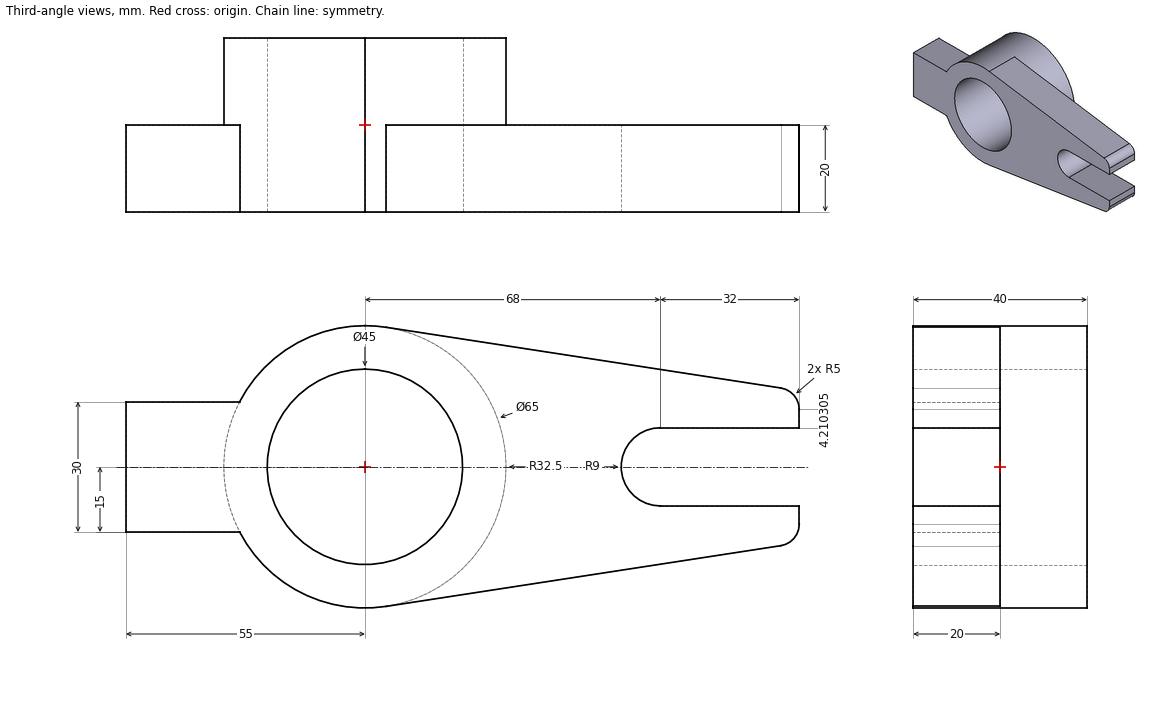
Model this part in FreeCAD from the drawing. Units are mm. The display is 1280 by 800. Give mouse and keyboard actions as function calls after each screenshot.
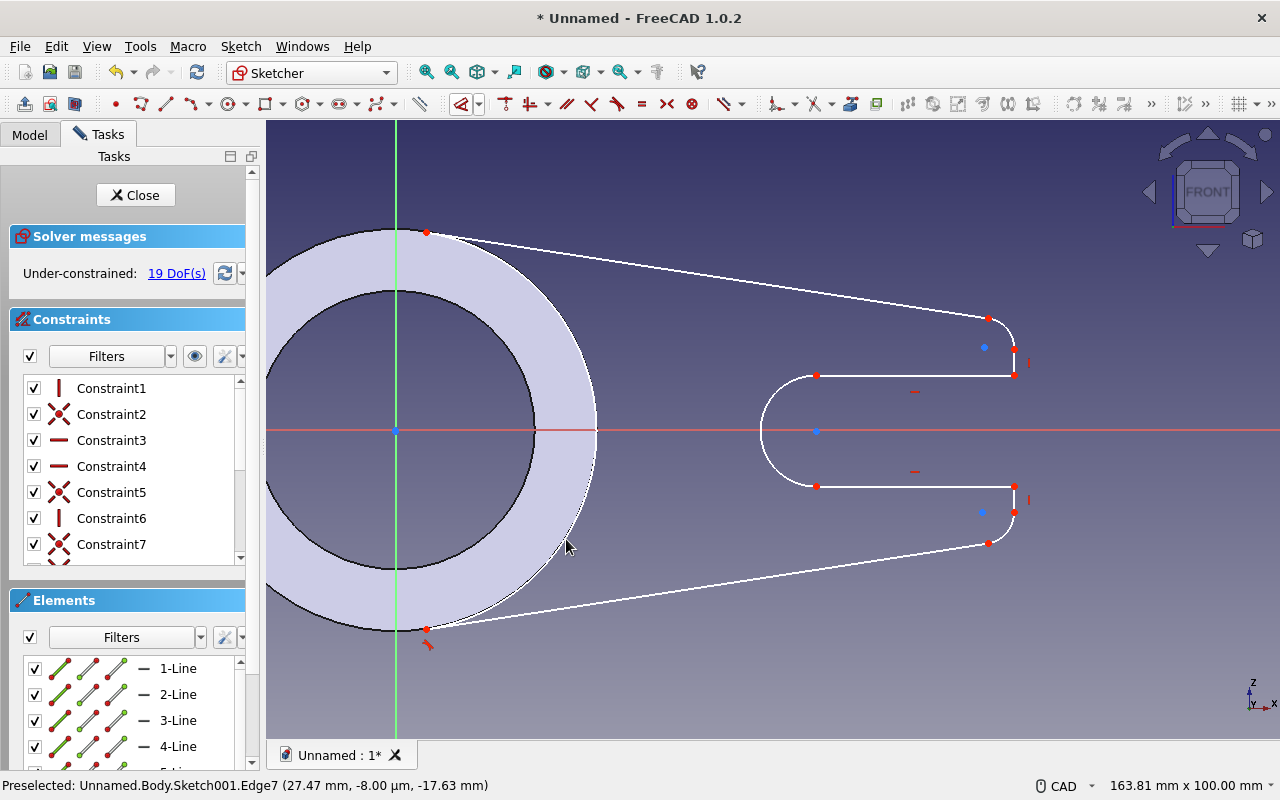
click(820, 569)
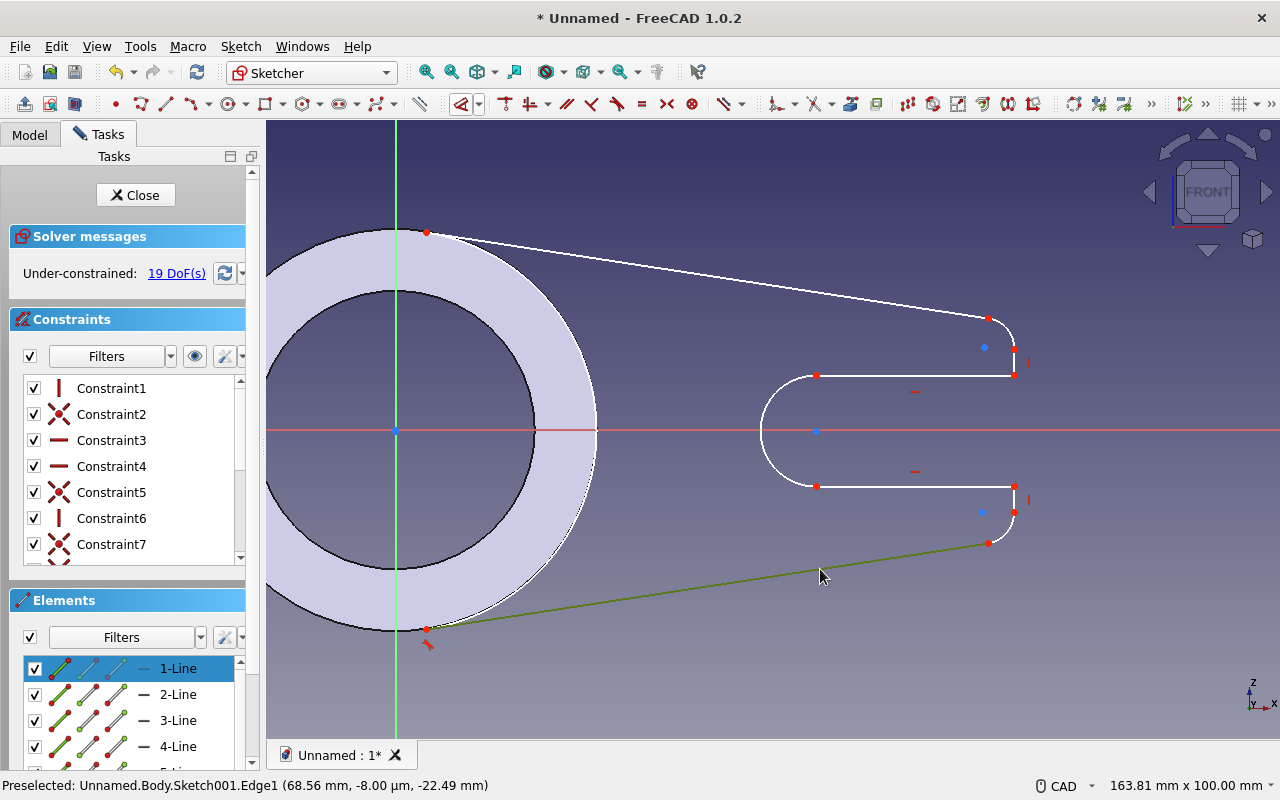
click(1000, 539)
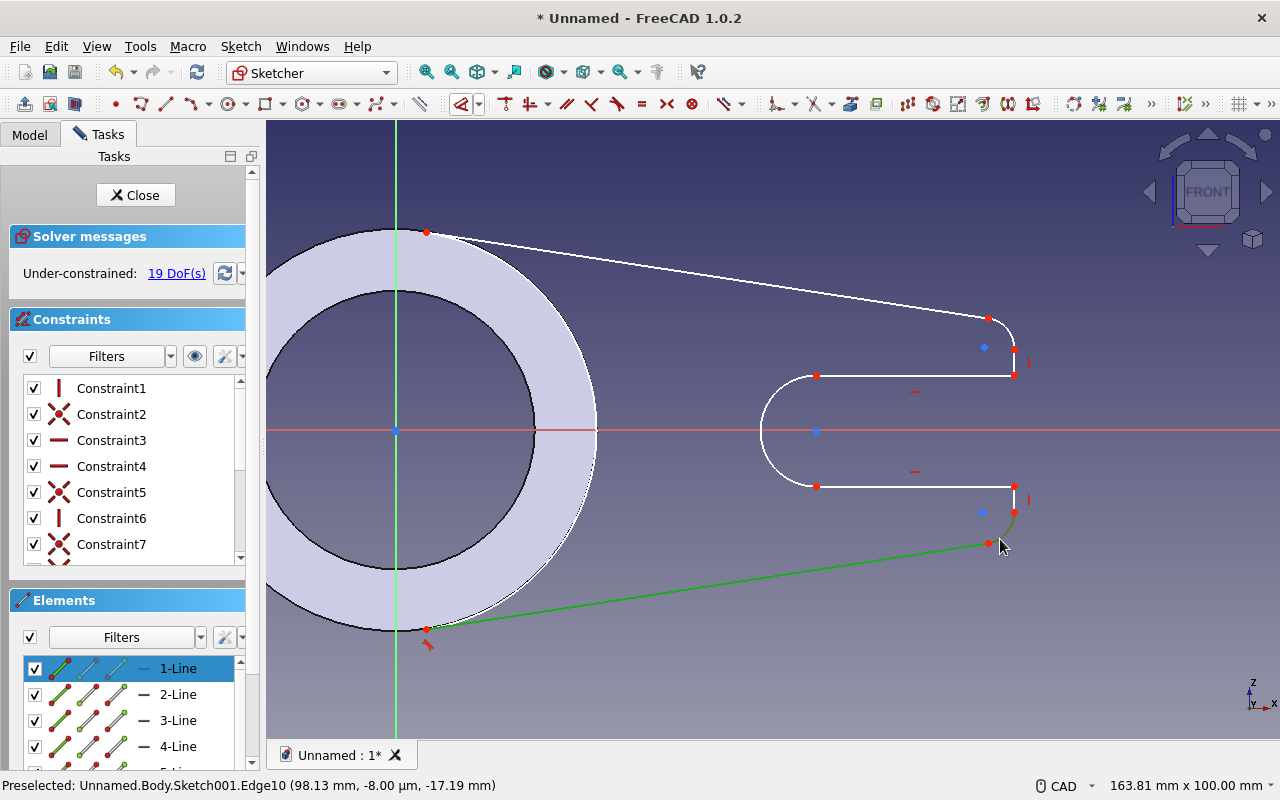
key(t)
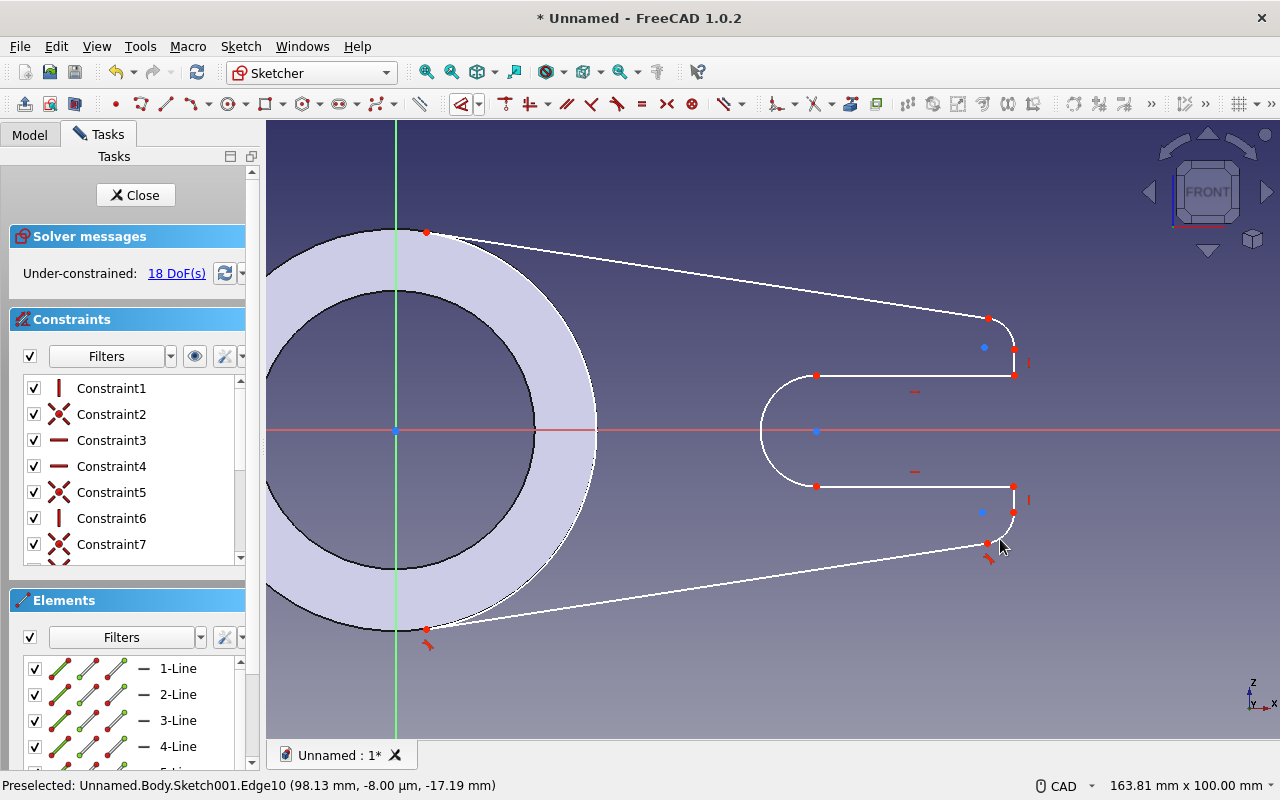
click(595, 258)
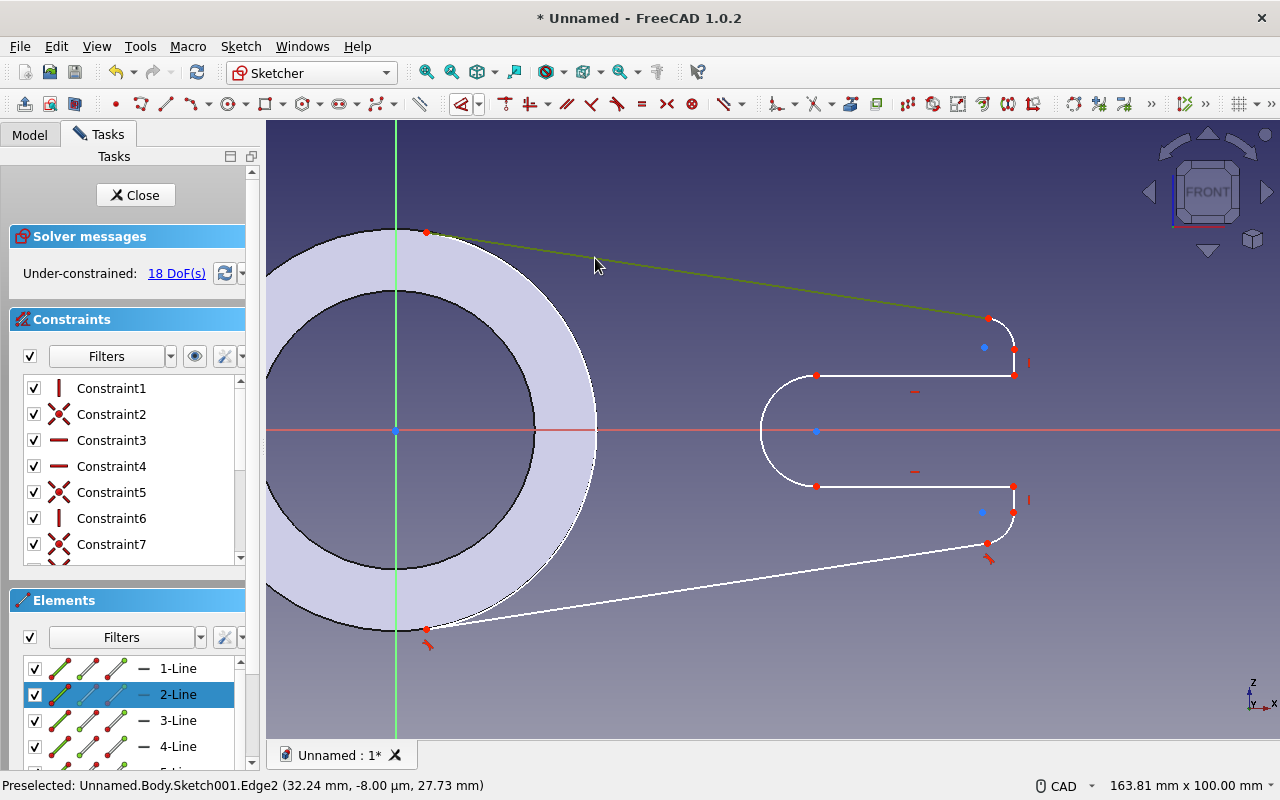
click(565, 539)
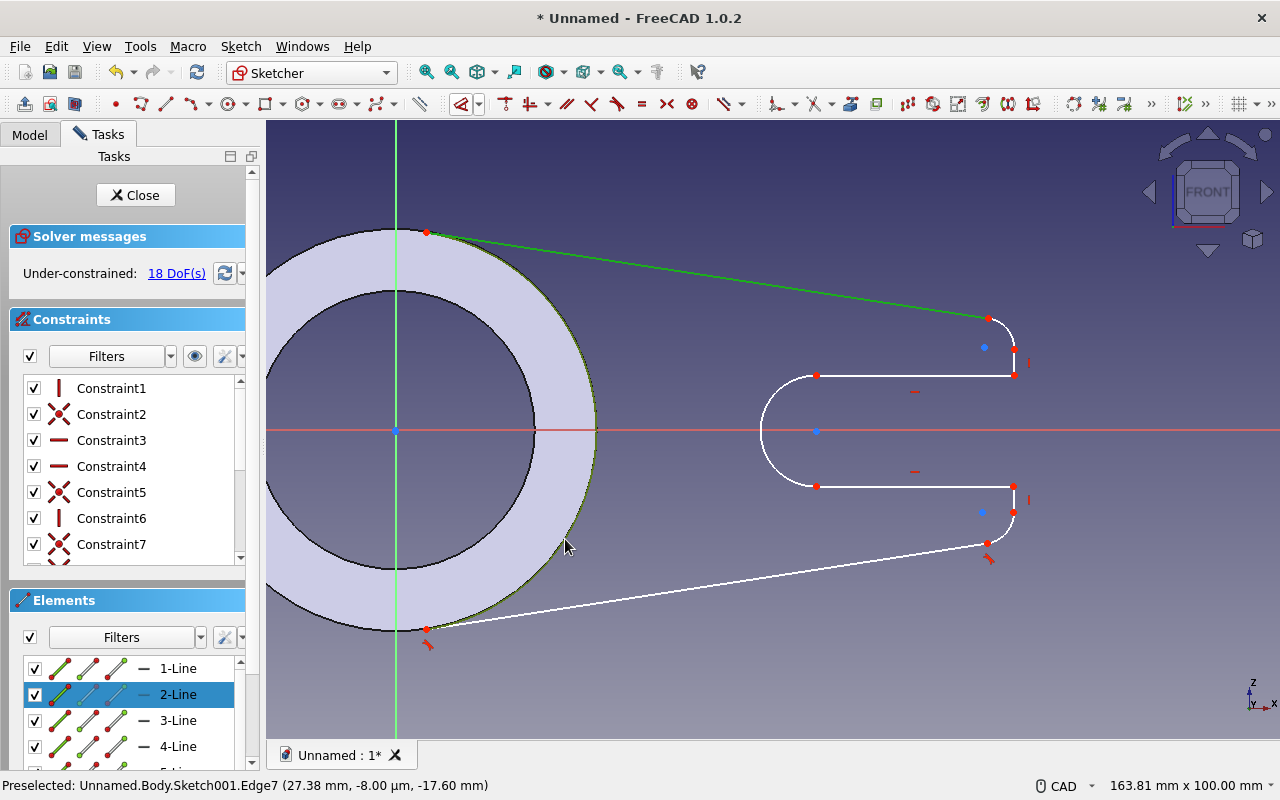
click(617, 104)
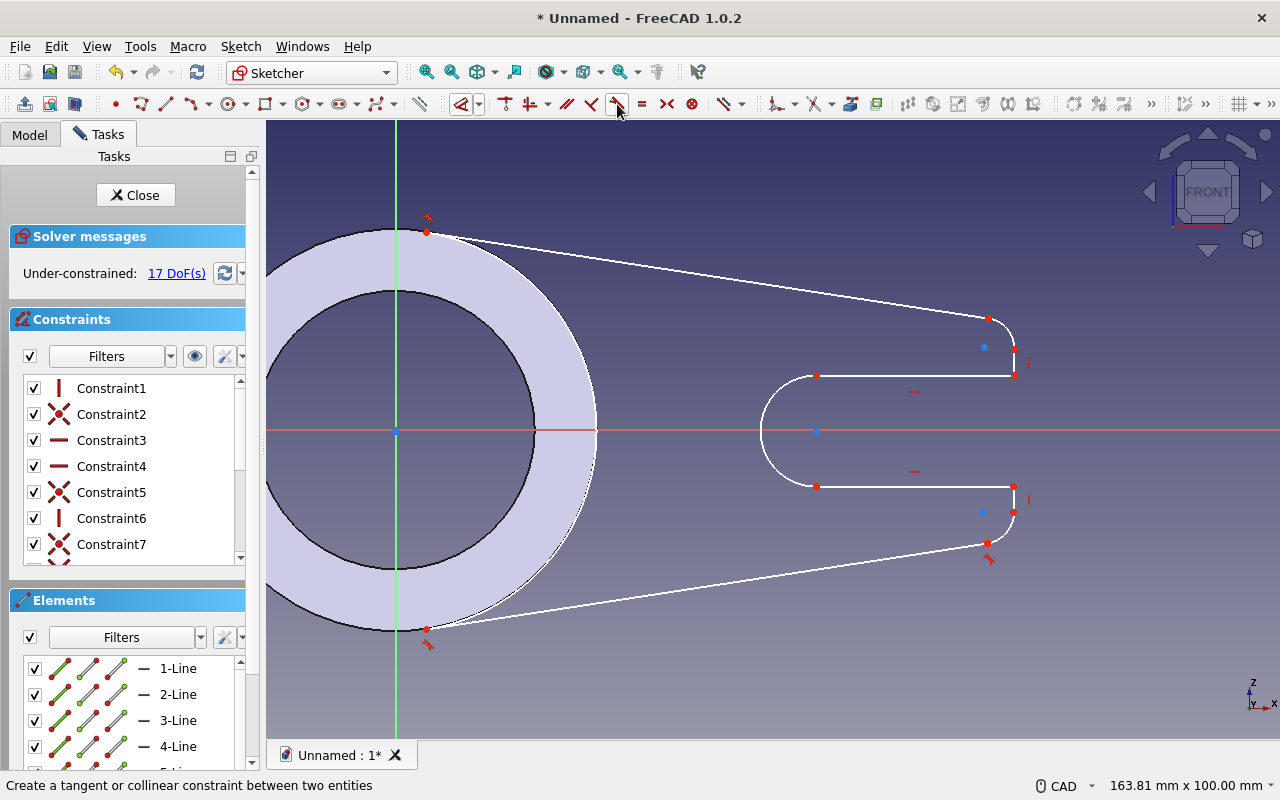
click(595, 258)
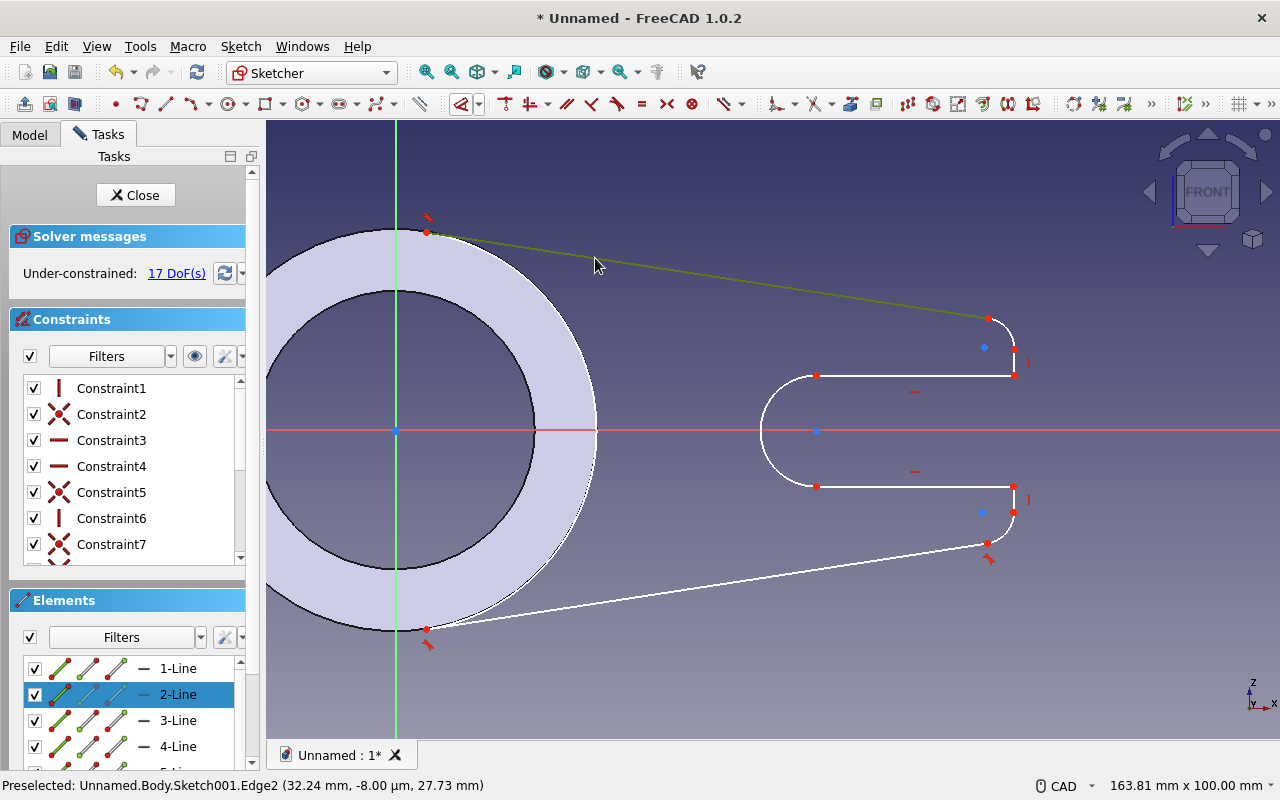
click(1012, 337)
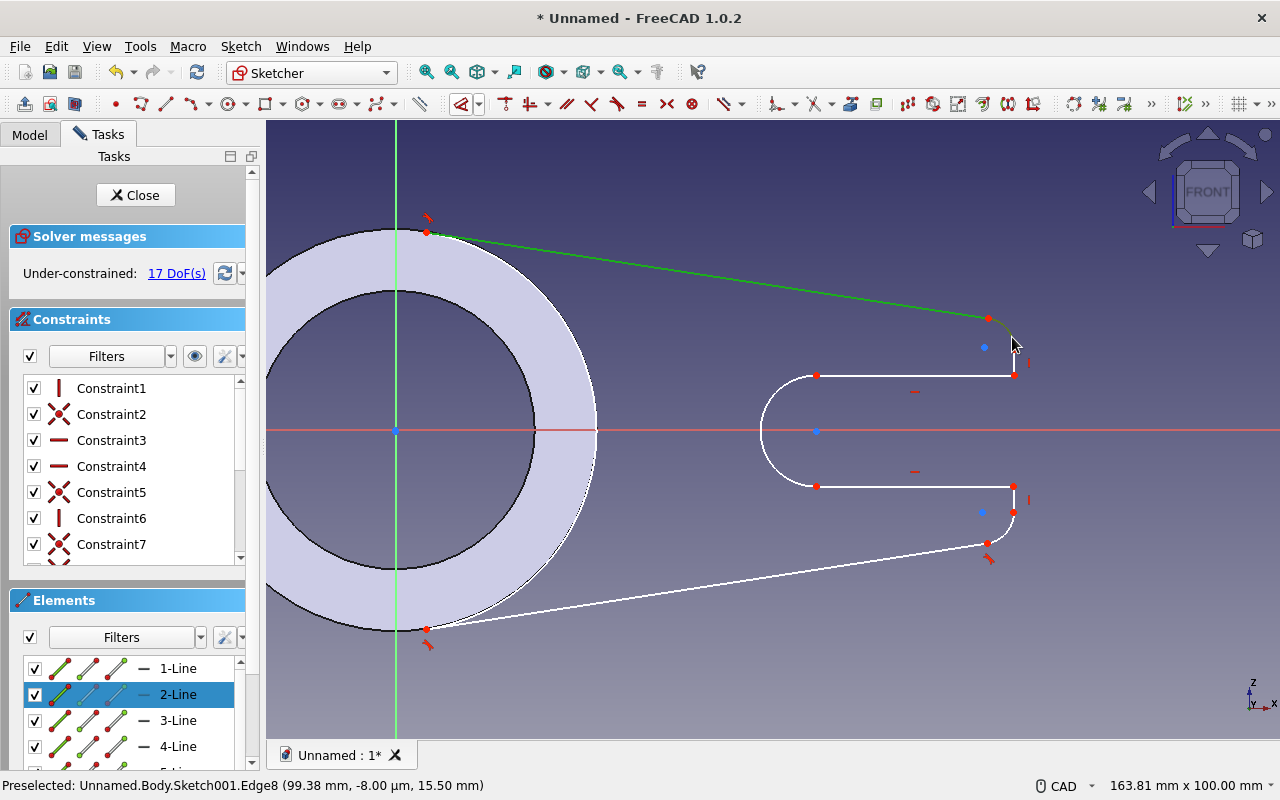
click(617, 104)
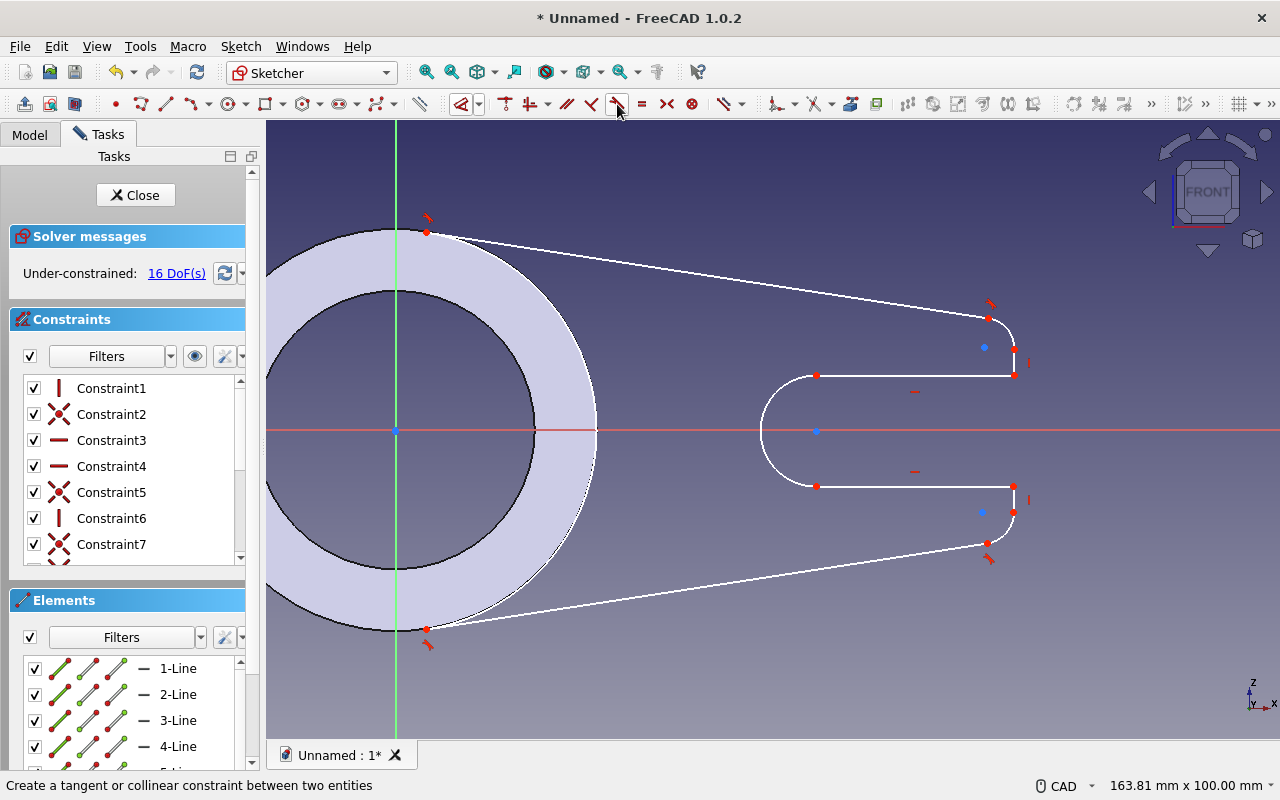
scroll(1014, 360, up, 2)